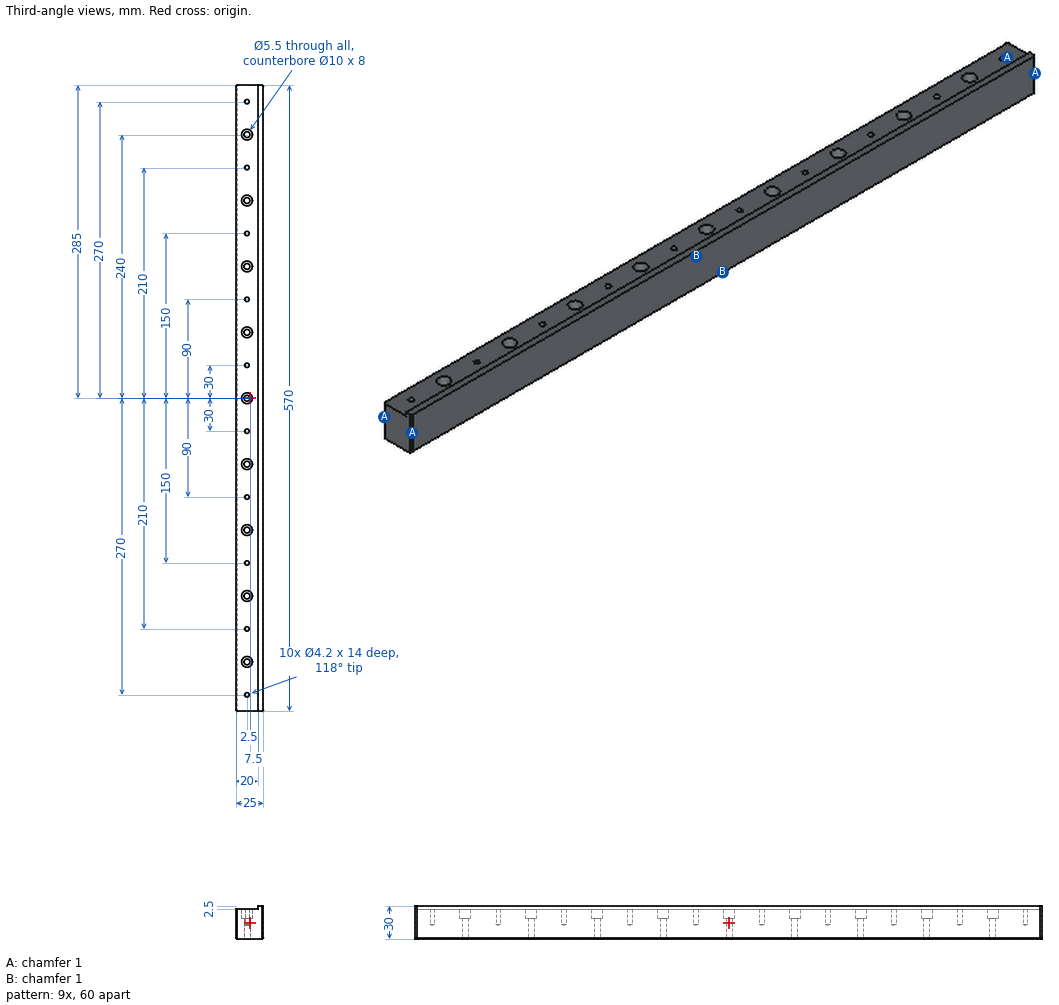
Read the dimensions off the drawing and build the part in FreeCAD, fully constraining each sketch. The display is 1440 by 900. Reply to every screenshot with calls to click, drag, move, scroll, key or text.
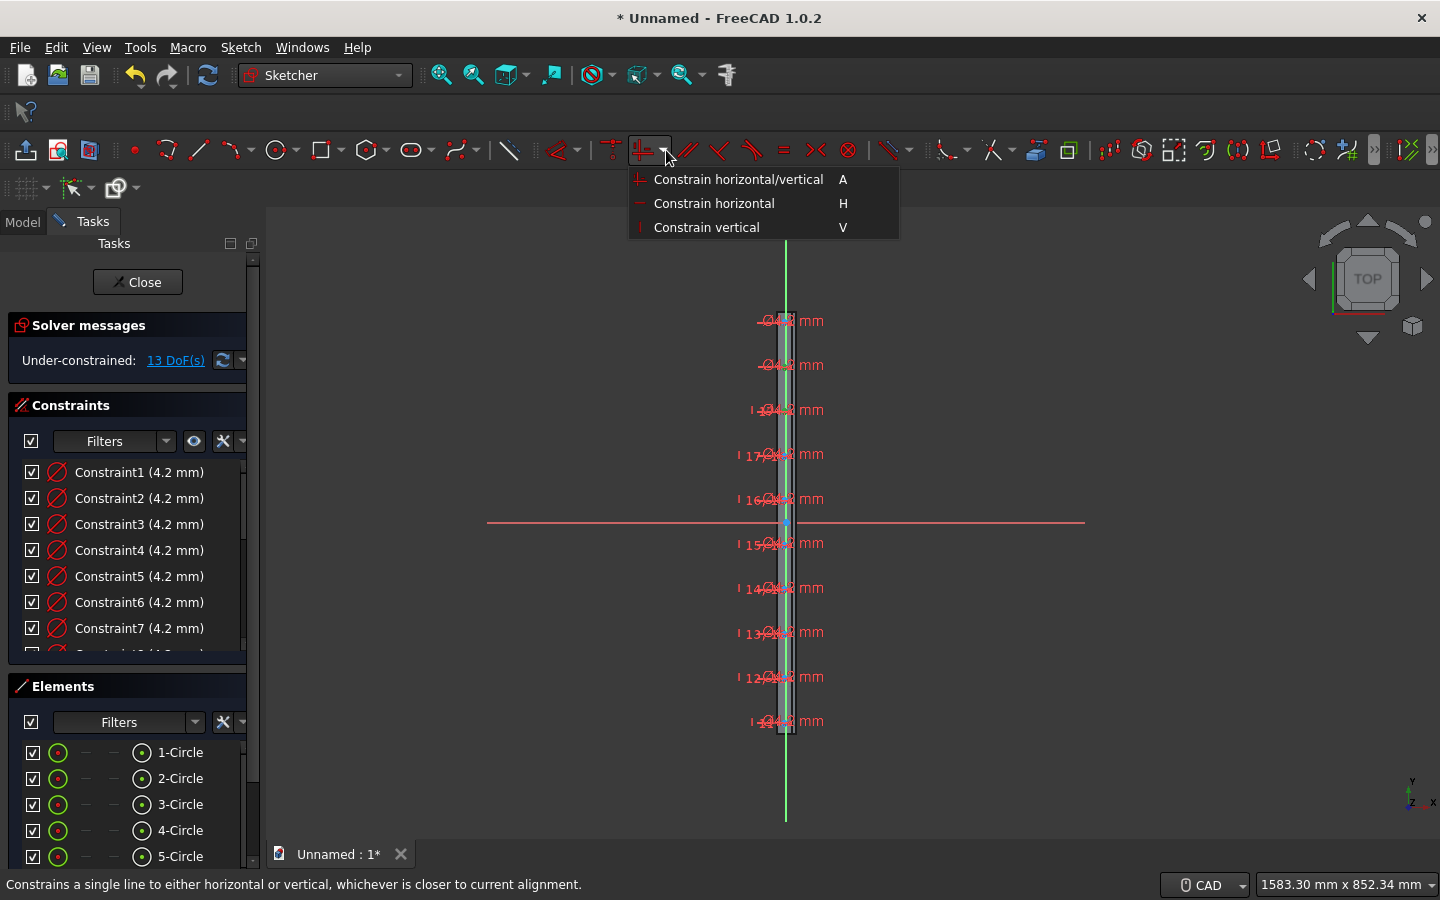
click(764, 227)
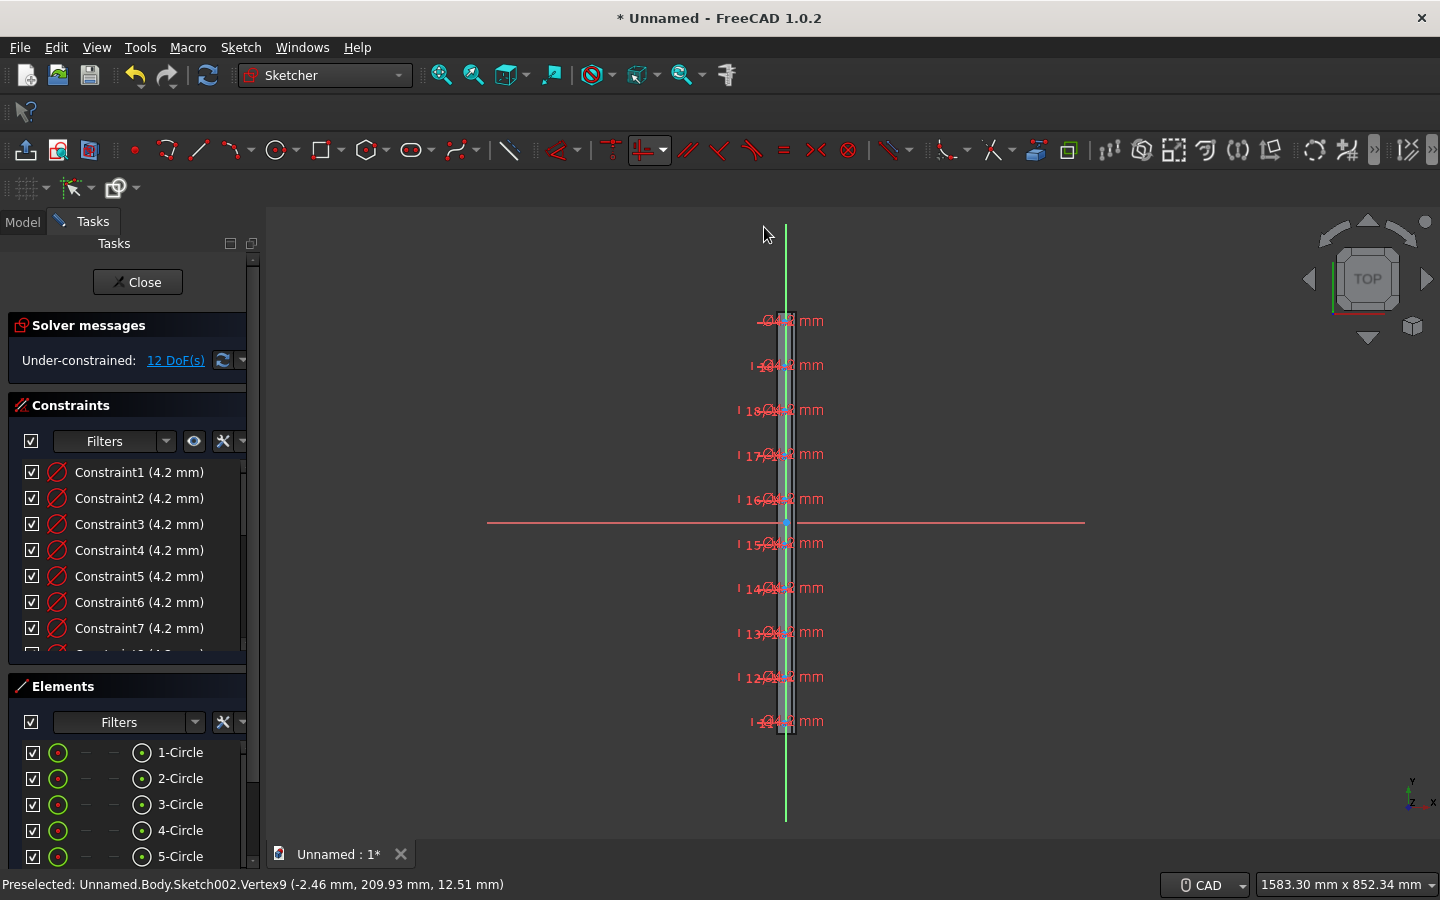
click(785, 367)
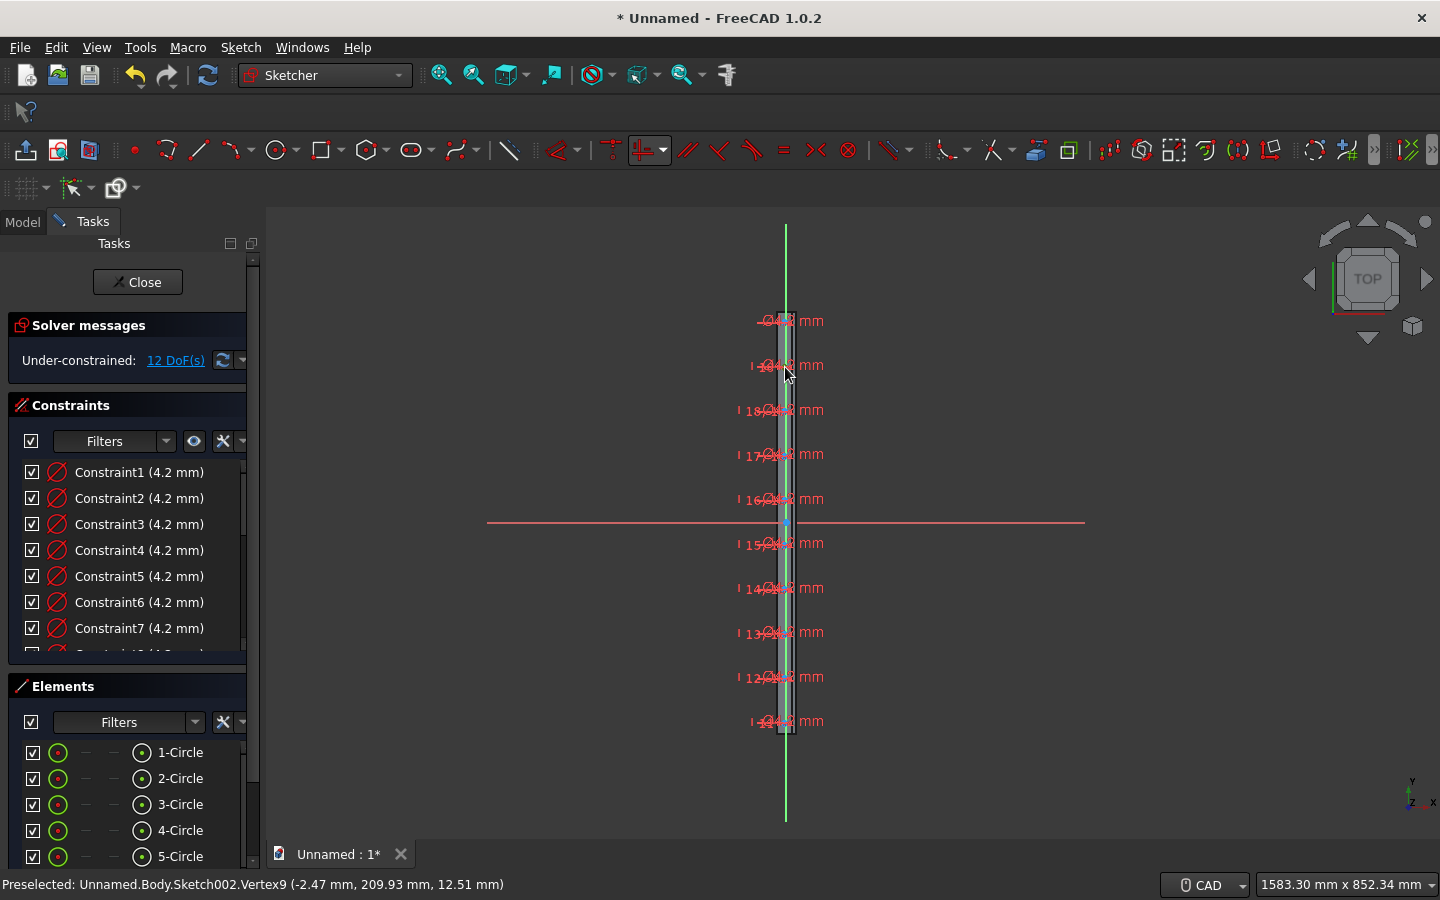
click(785, 323)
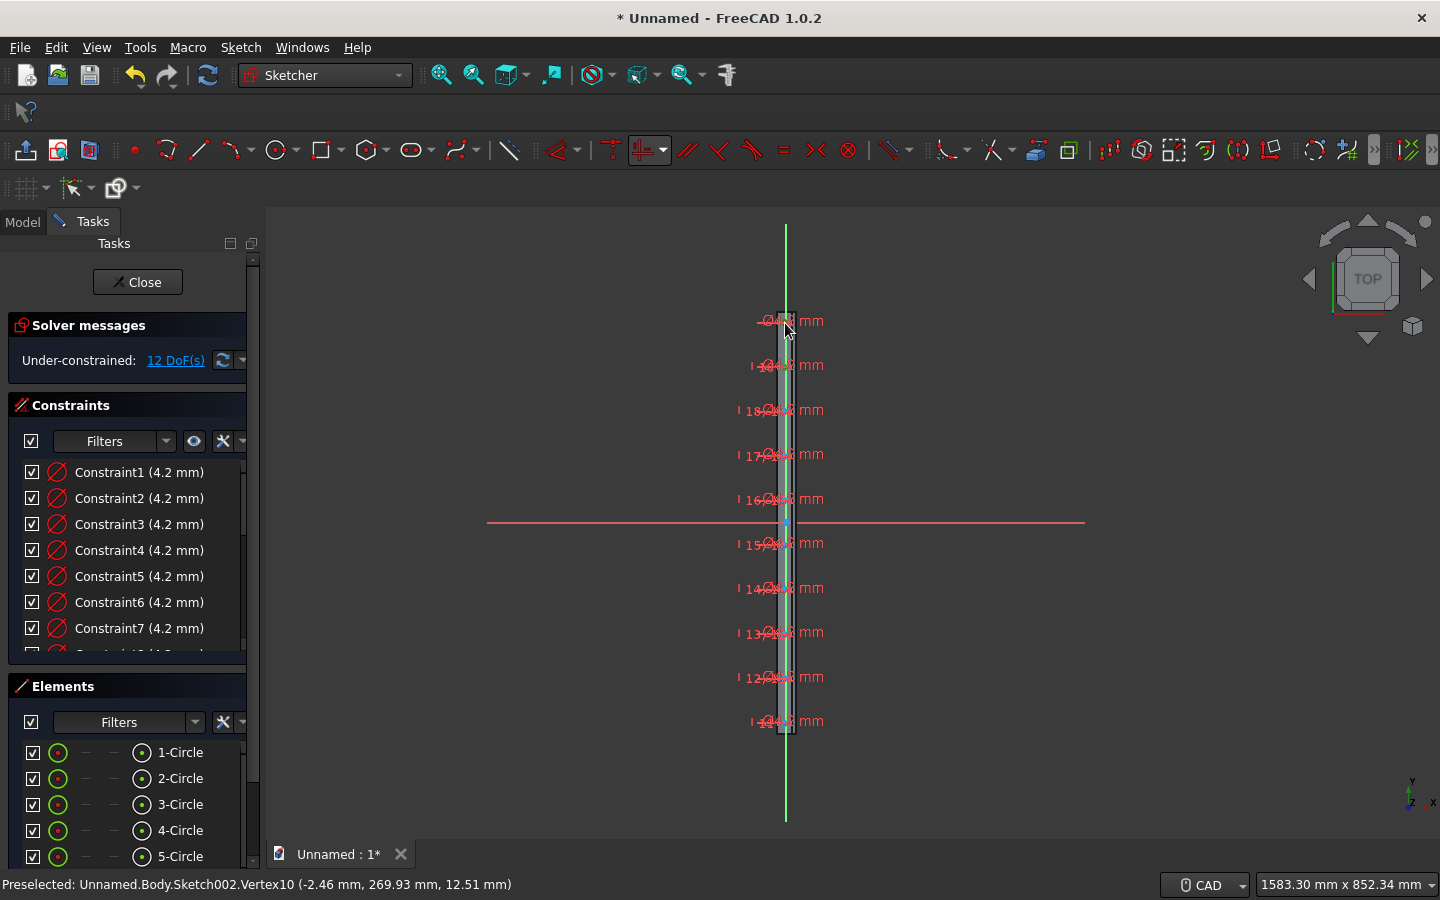
key(v)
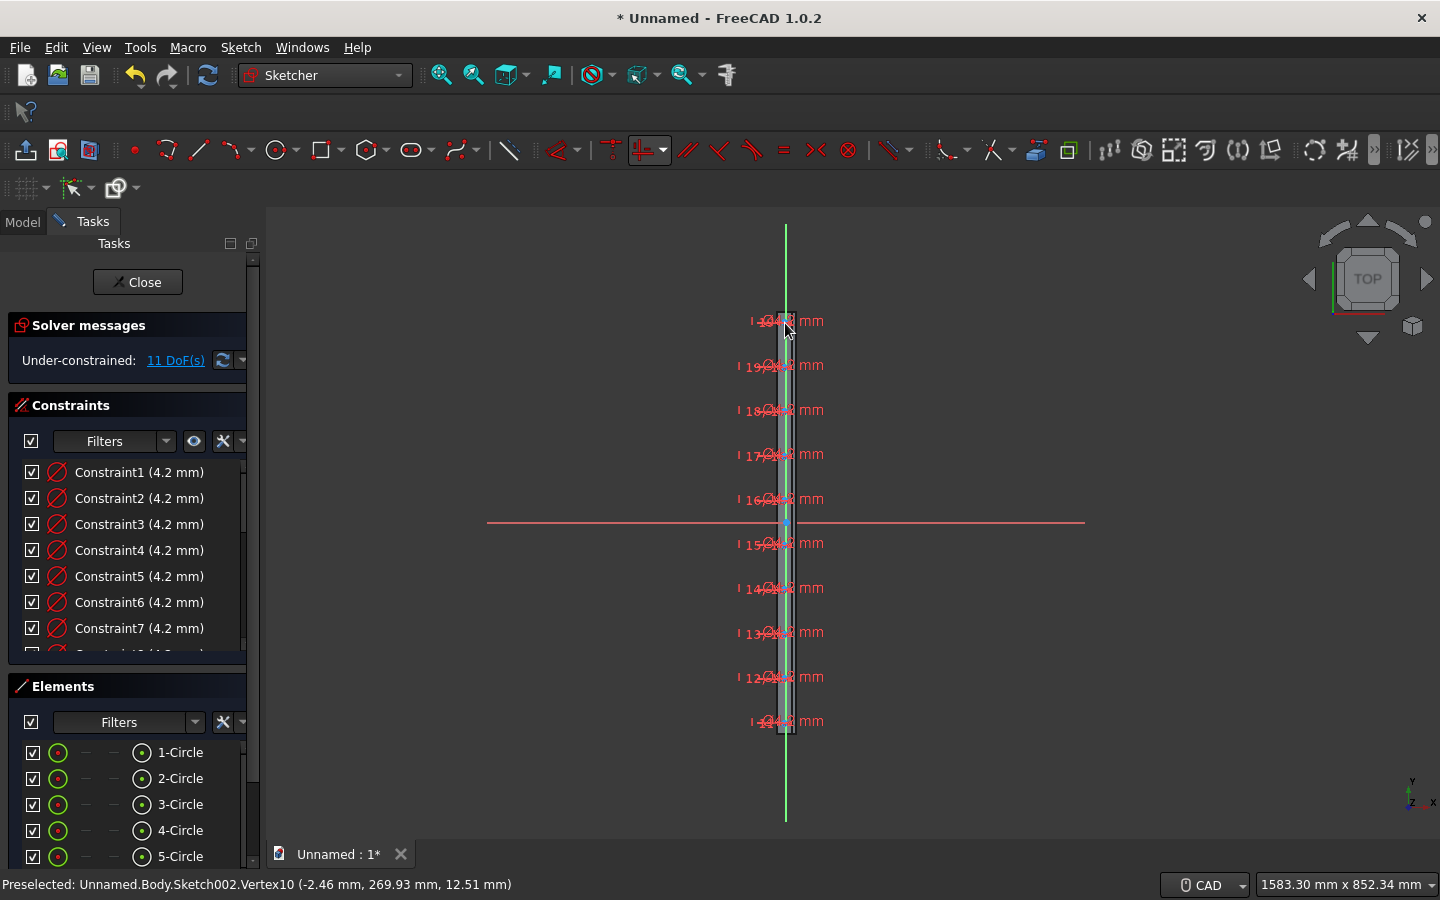
click(556, 150)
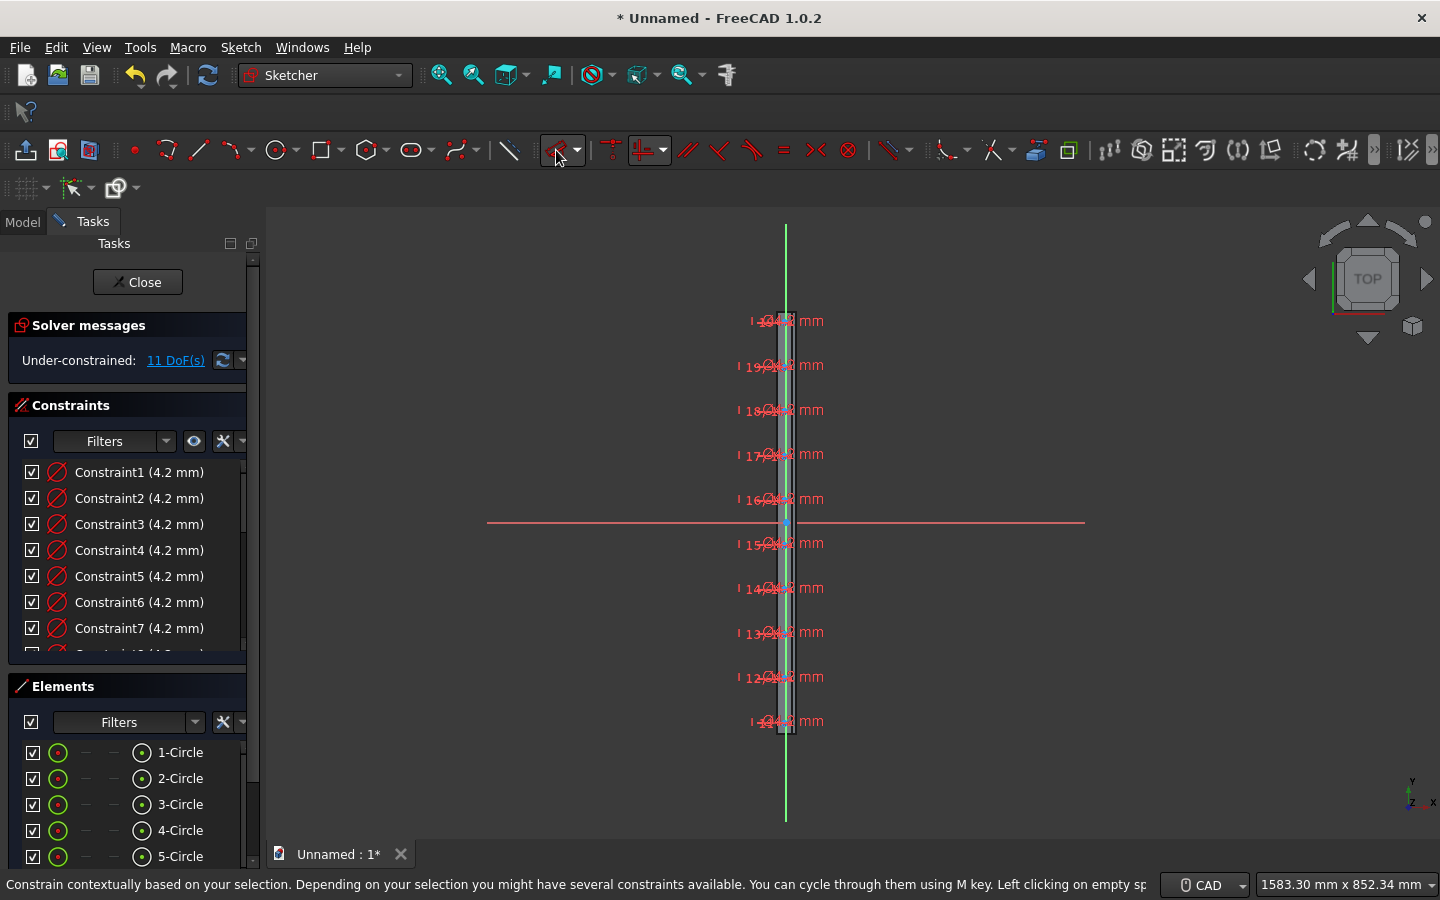
click(785, 590)
click(820, 556)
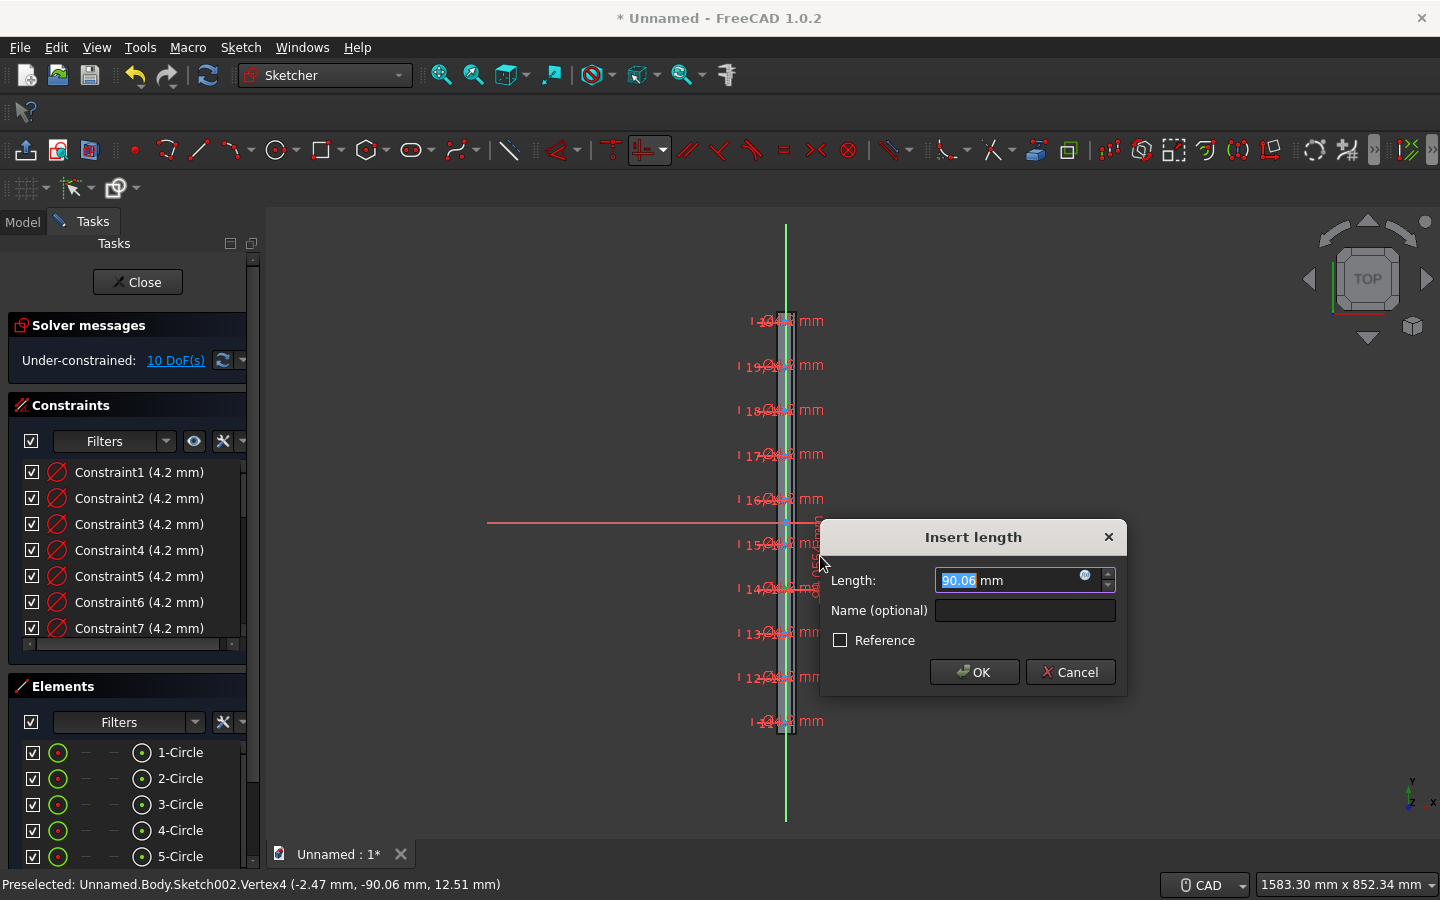
text(90)
key(Return)